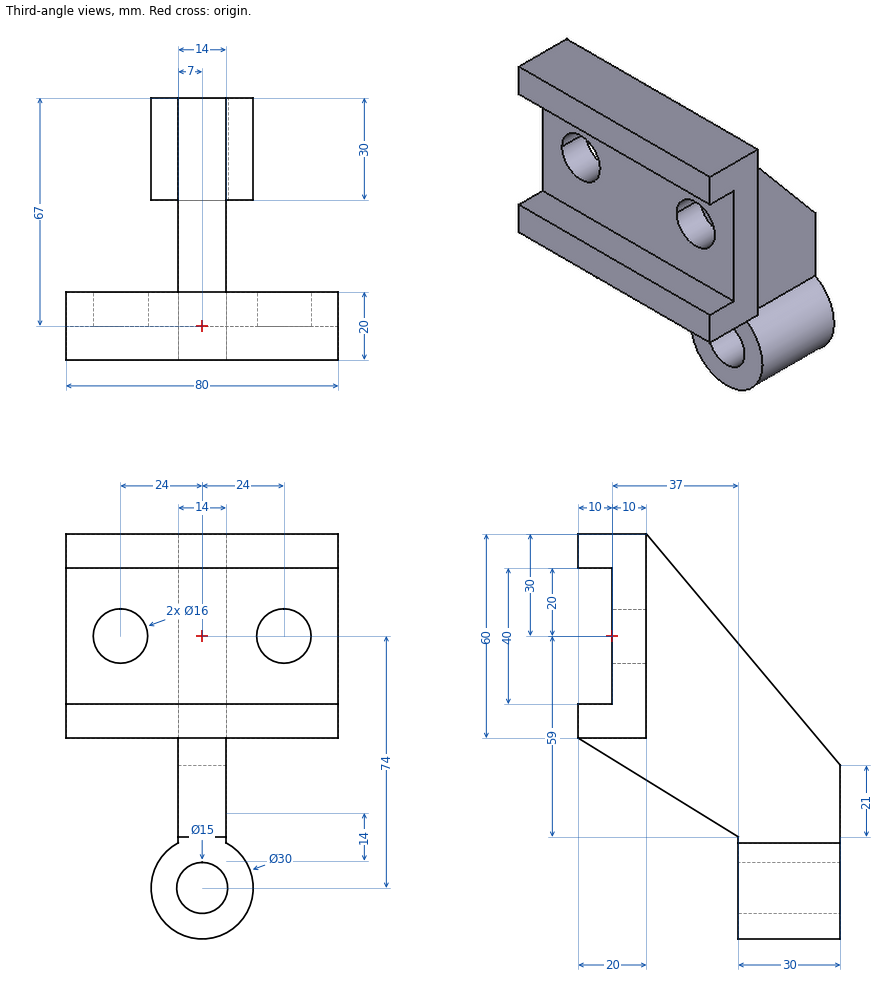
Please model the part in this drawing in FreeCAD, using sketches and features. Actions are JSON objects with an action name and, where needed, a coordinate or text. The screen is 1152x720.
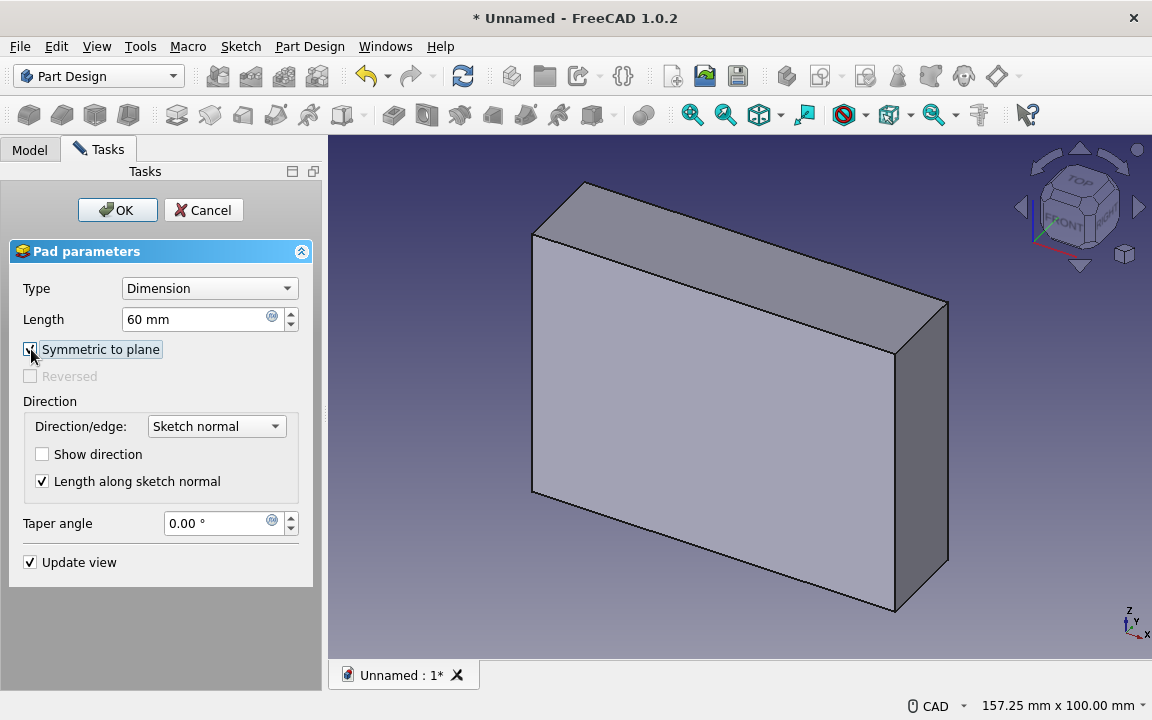
{"action": "left_click", "coordinate": [118, 210]}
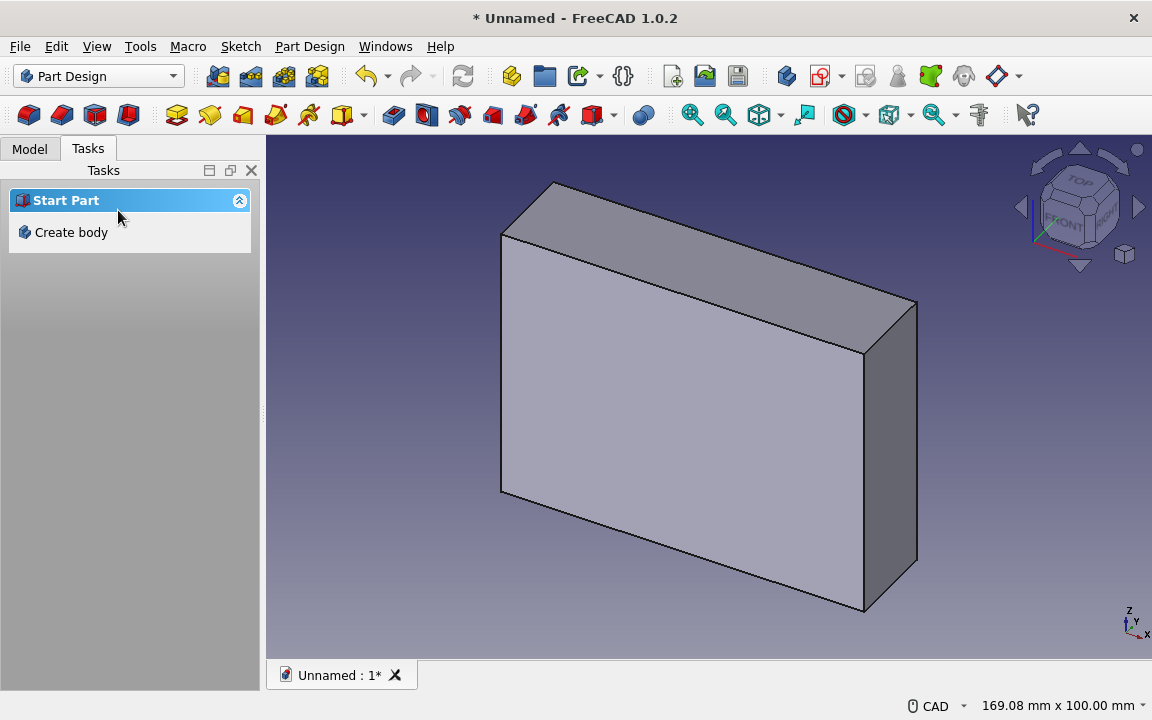
{"action": "left_click", "coordinate": [820, 76]}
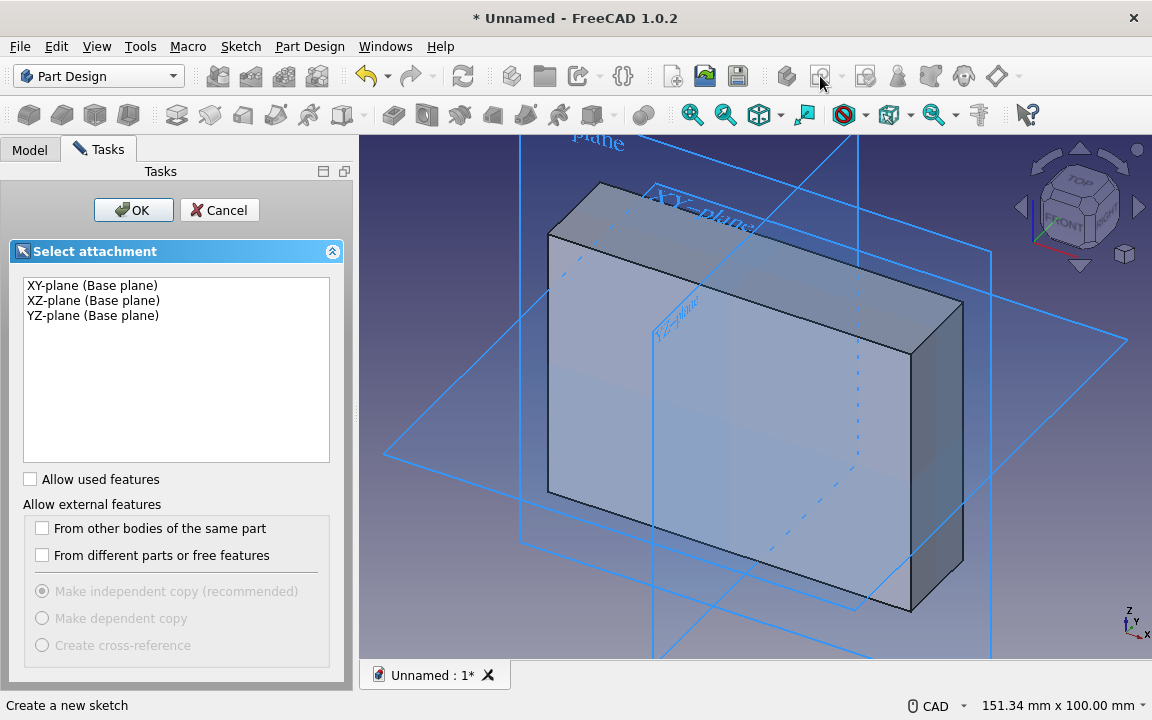
{"action": "left_click", "coordinate": [84, 316]}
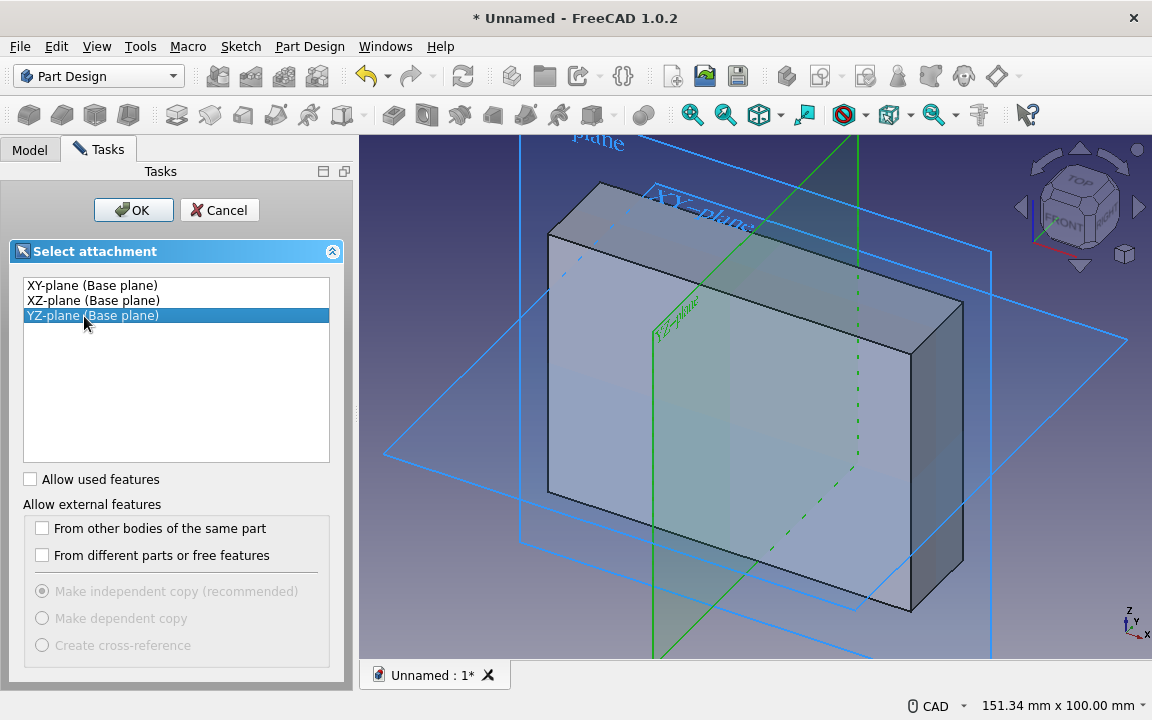
{"action": "left_click", "coordinate": [134, 210]}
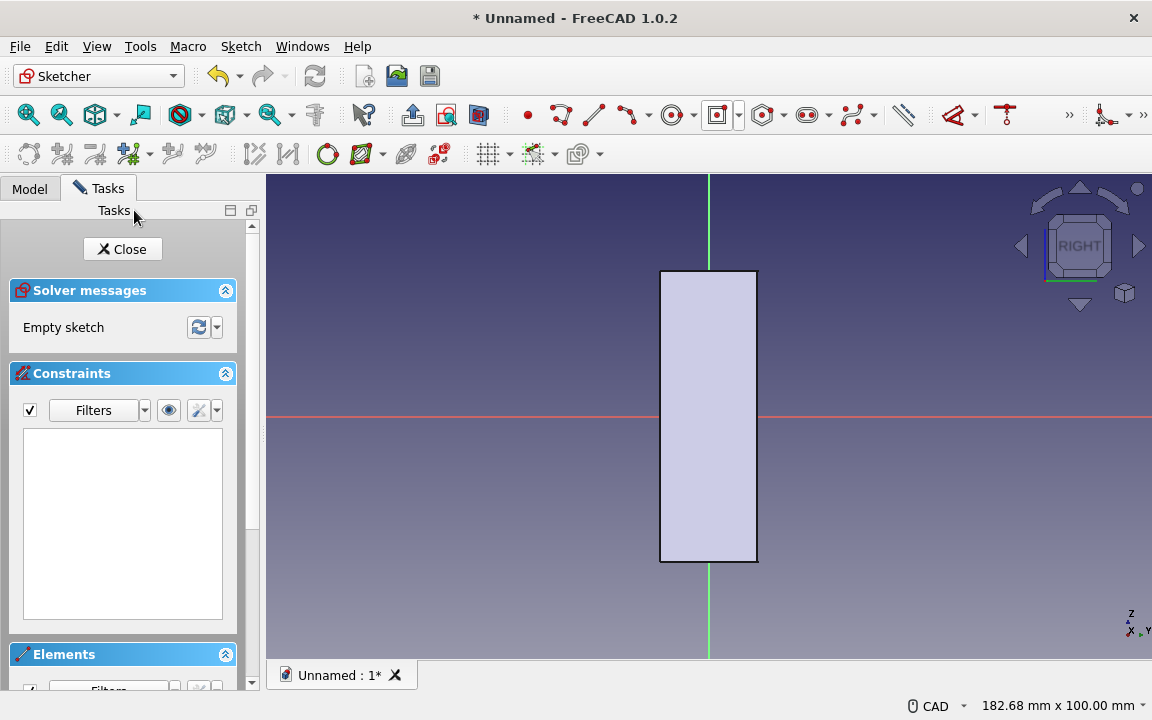
{"action": "left_click", "coordinate": [479, 116]}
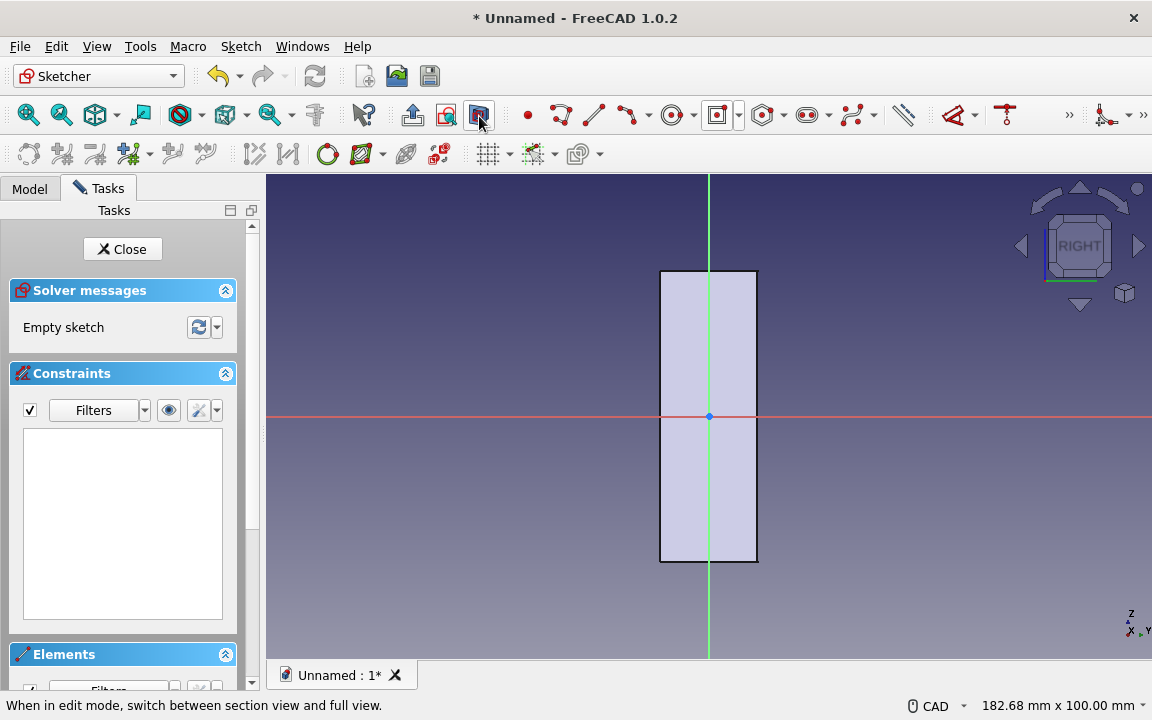
{"action": "scroll", "coordinate": [294, 274], "scroll_direction": "down", "scroll_amount": 2}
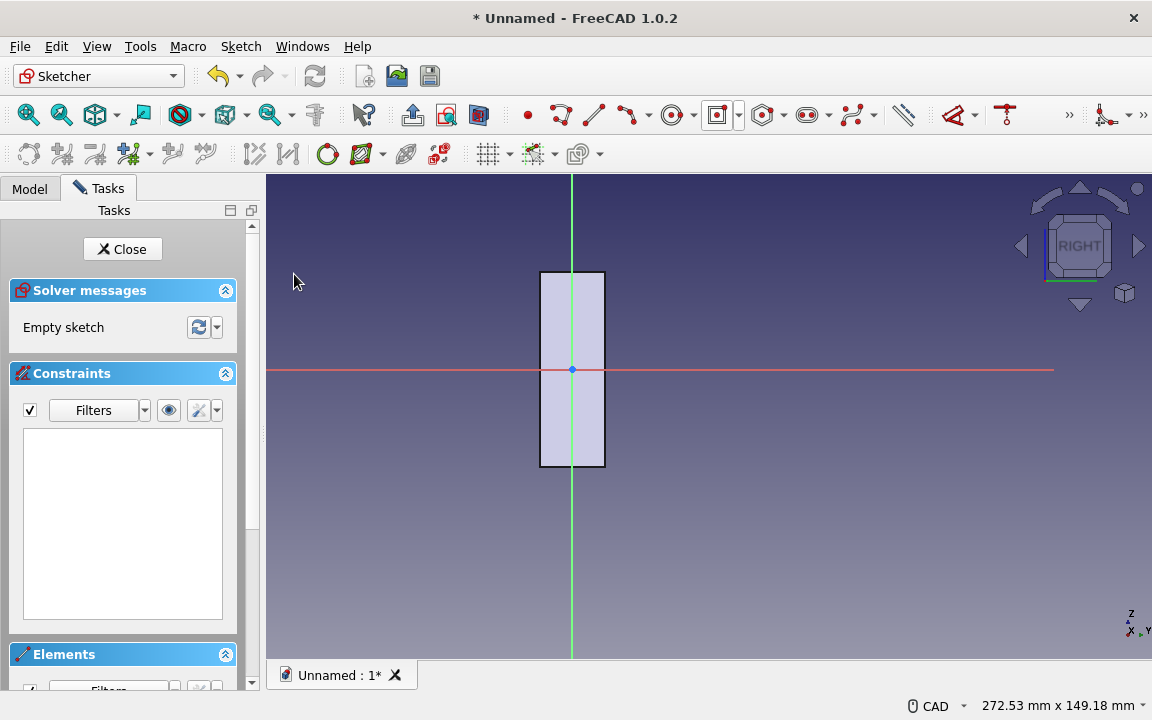
{"action": "left_click", "coordinate": [561, 116]}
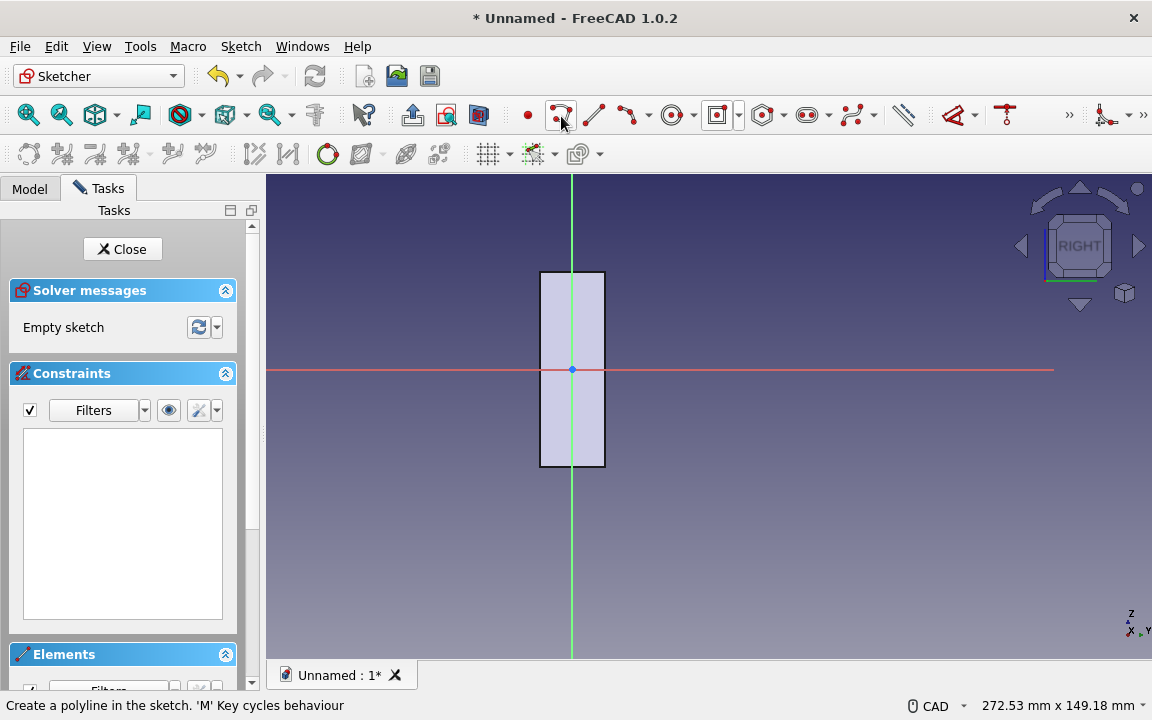
{"action": "left_click", "coordinate": [605, 272]}
{"action": "left_click", "coordinate": [605, 467]}
{"action": "left_click", "coordinate": [540, 467]}
{"action": "left_click", "coordinate": [692, 561]}
{"action": "left_click", "coordinate": [790, 561]}
{"action": "left_click", "coordinate": [790, 493]}
{"action": "left_click", "coordinate": [605, 273]}
{"action": "key", "text": "Escape"}
{"action": "key", "text": "Escape"}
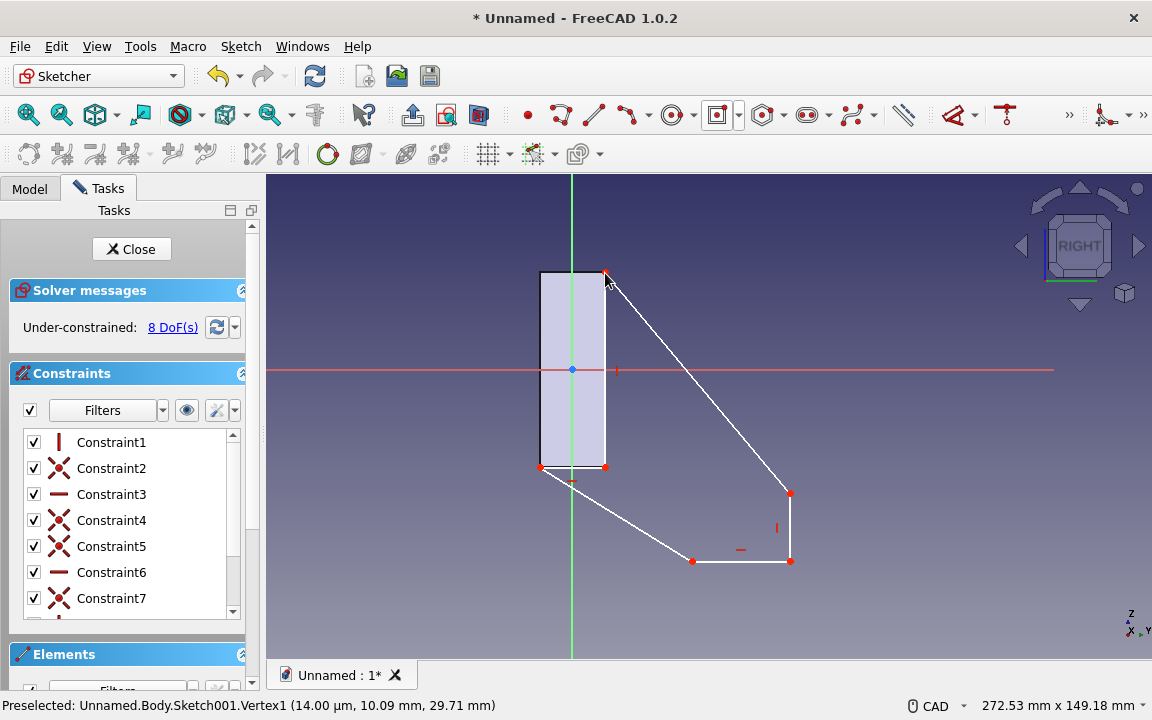
{"action": "left_click", "coordinate": [605, 332]}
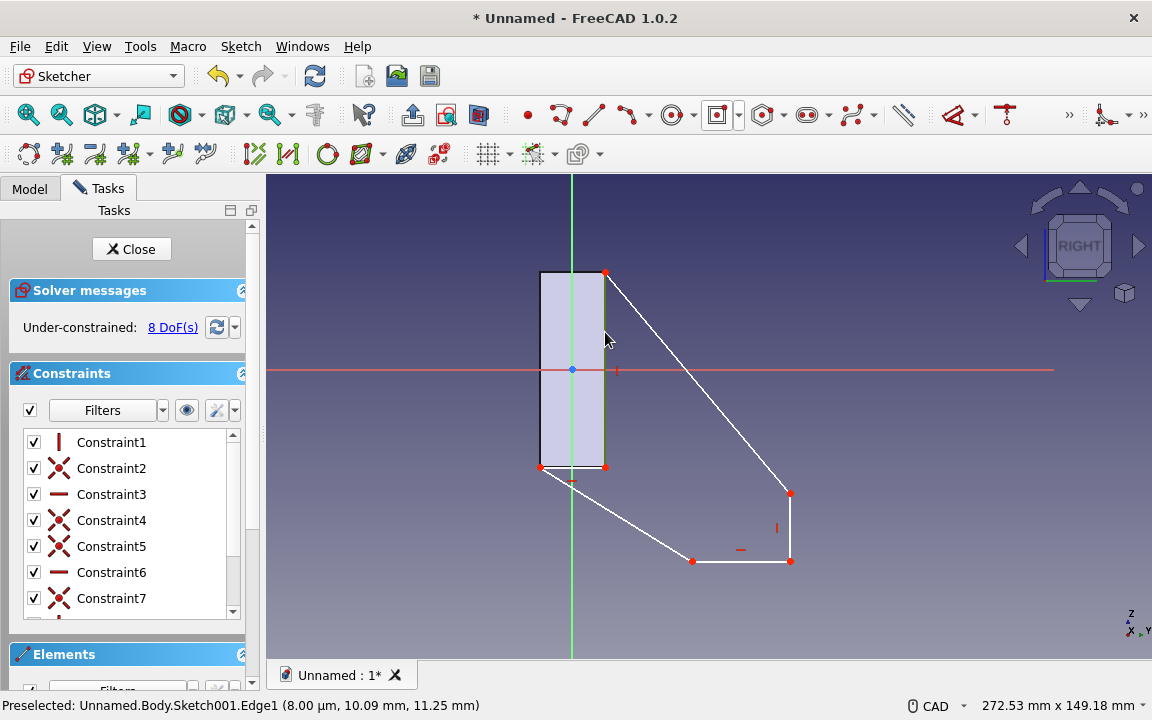
{"action": "key", "text": "i"}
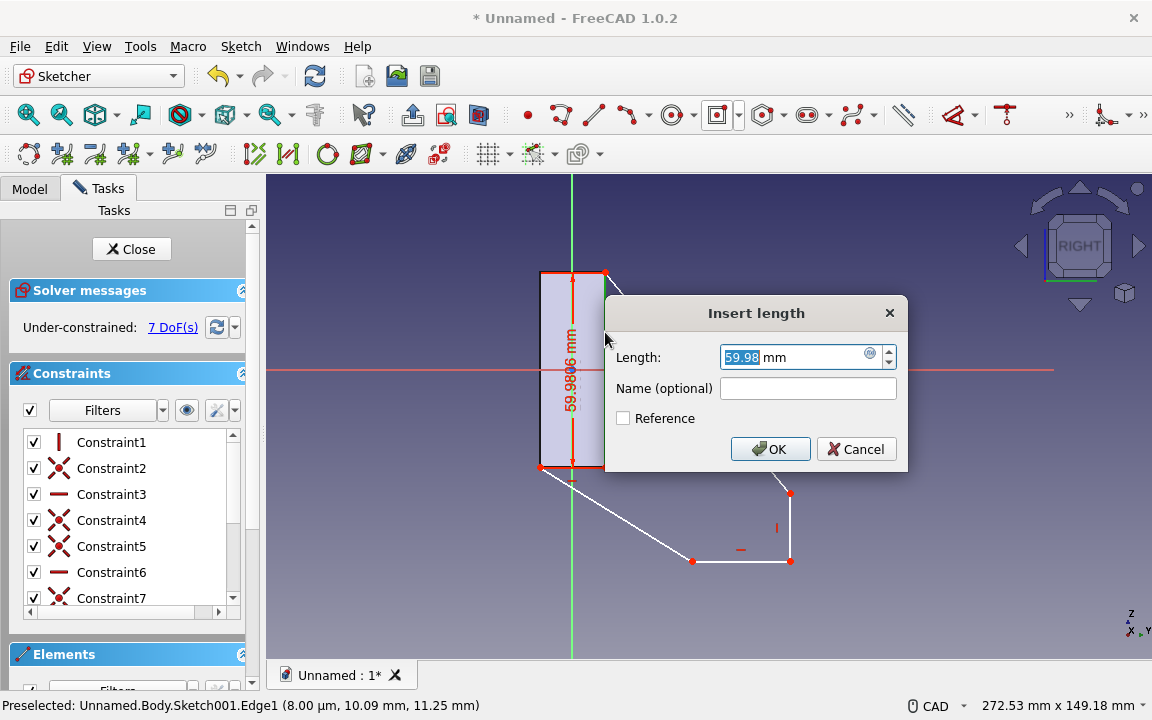
{"action": "type", "text": "60"}
{"action": "key", "text": "Return"}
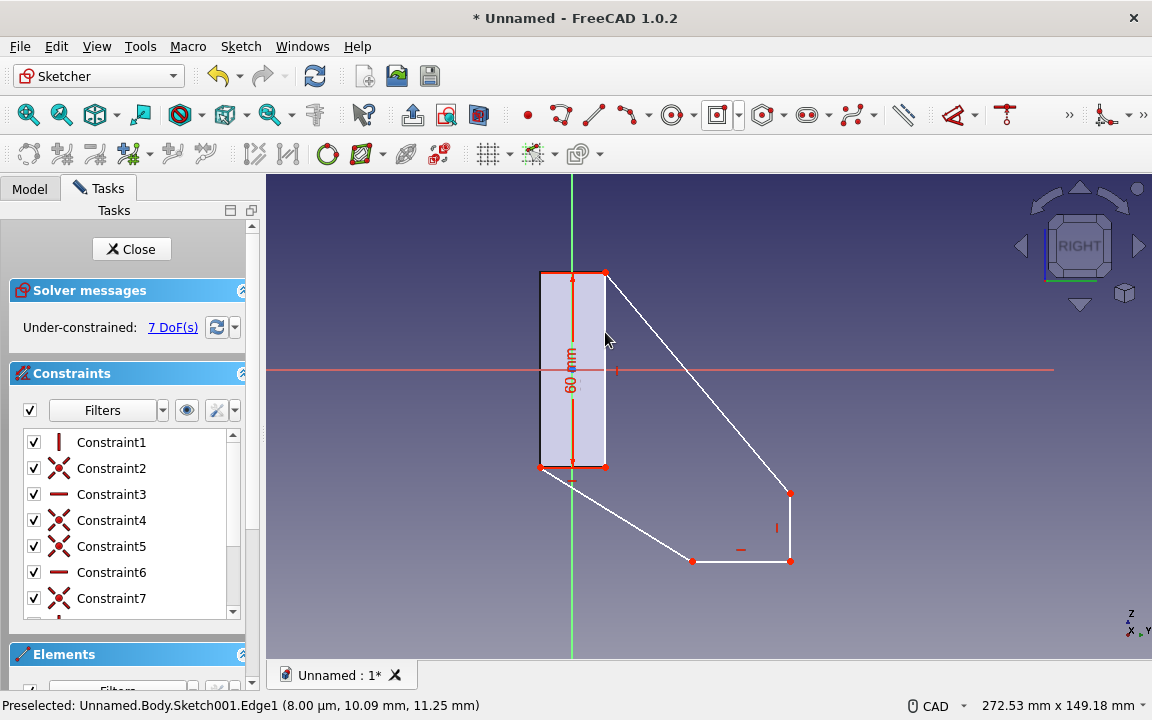
{"action": "left_click", "coordinate": [586, 468]}